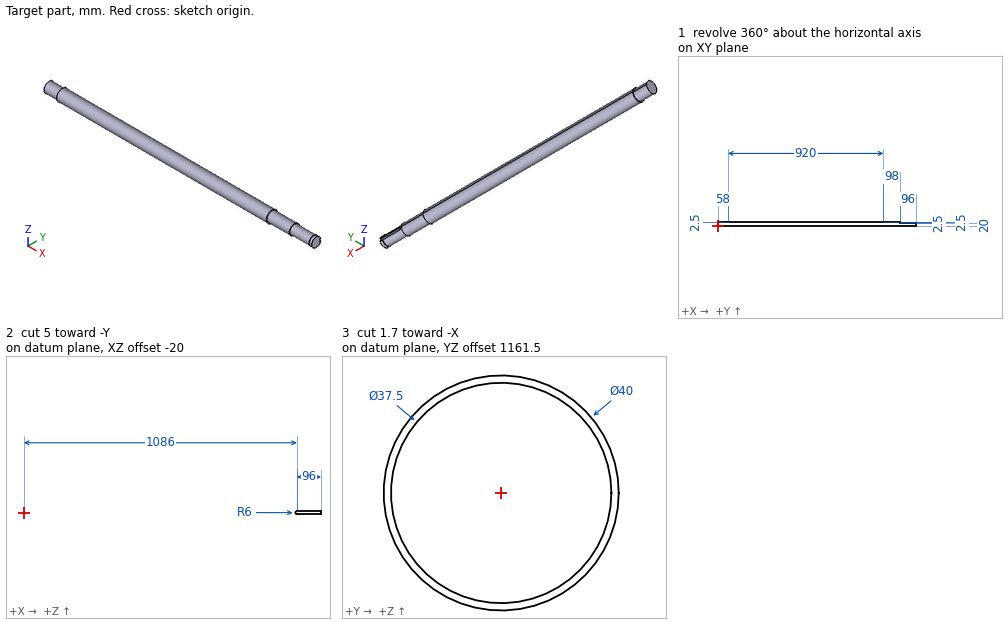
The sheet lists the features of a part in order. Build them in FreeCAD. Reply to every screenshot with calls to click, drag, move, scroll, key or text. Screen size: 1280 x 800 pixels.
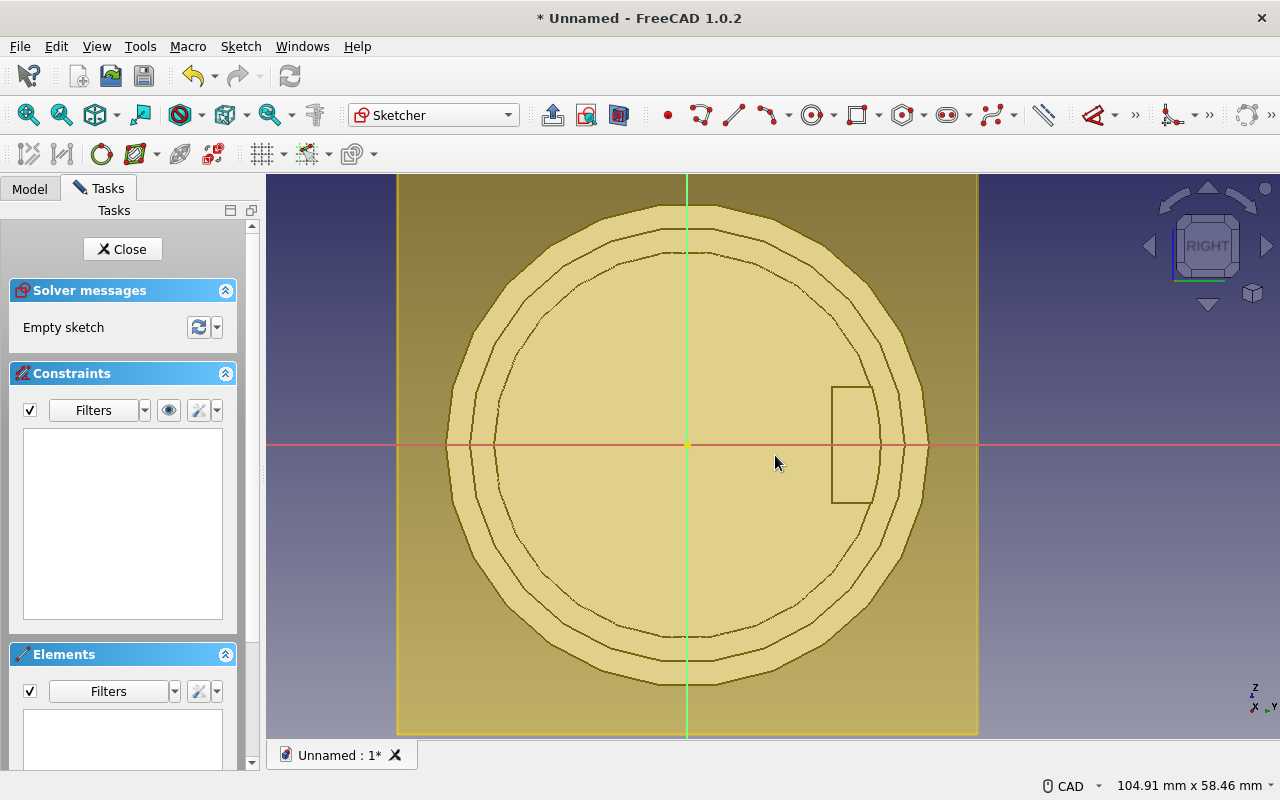
click(812, 116)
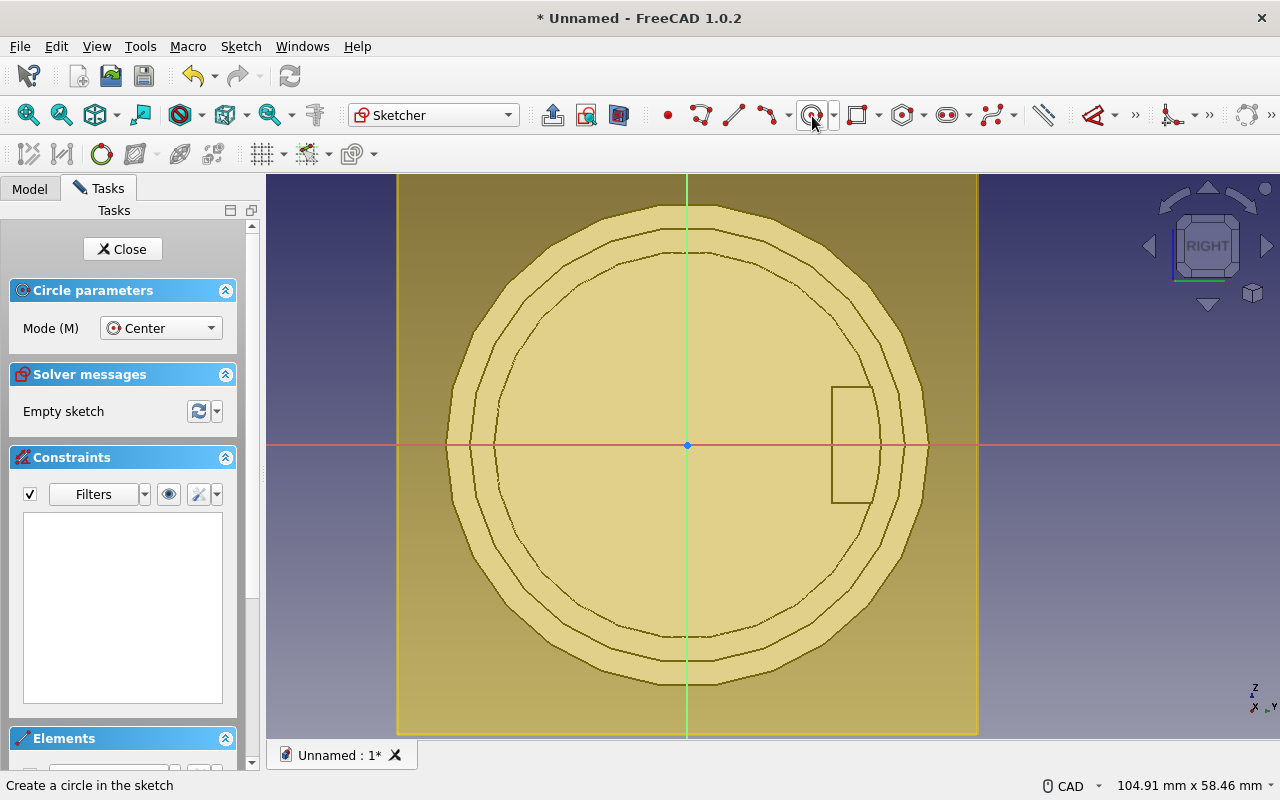
click(687, 445)
click(824, 308)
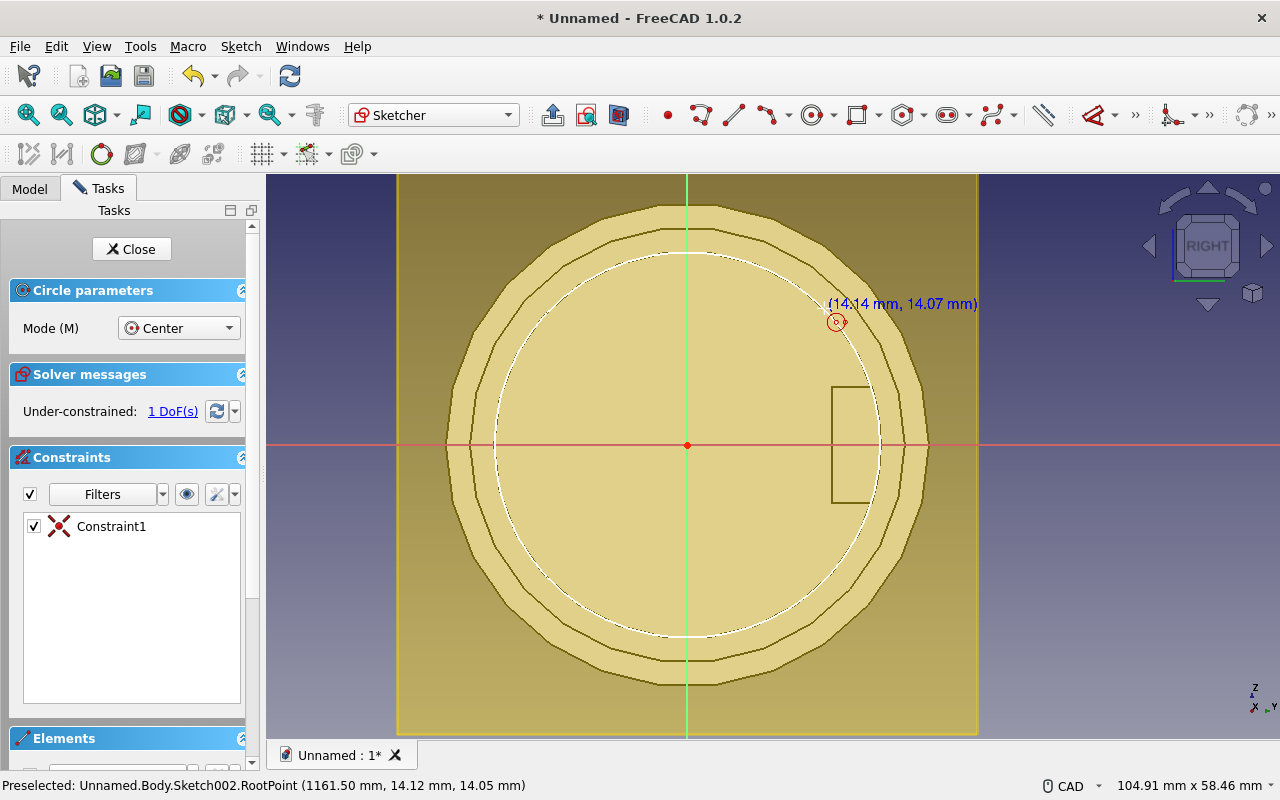
click(687, 445)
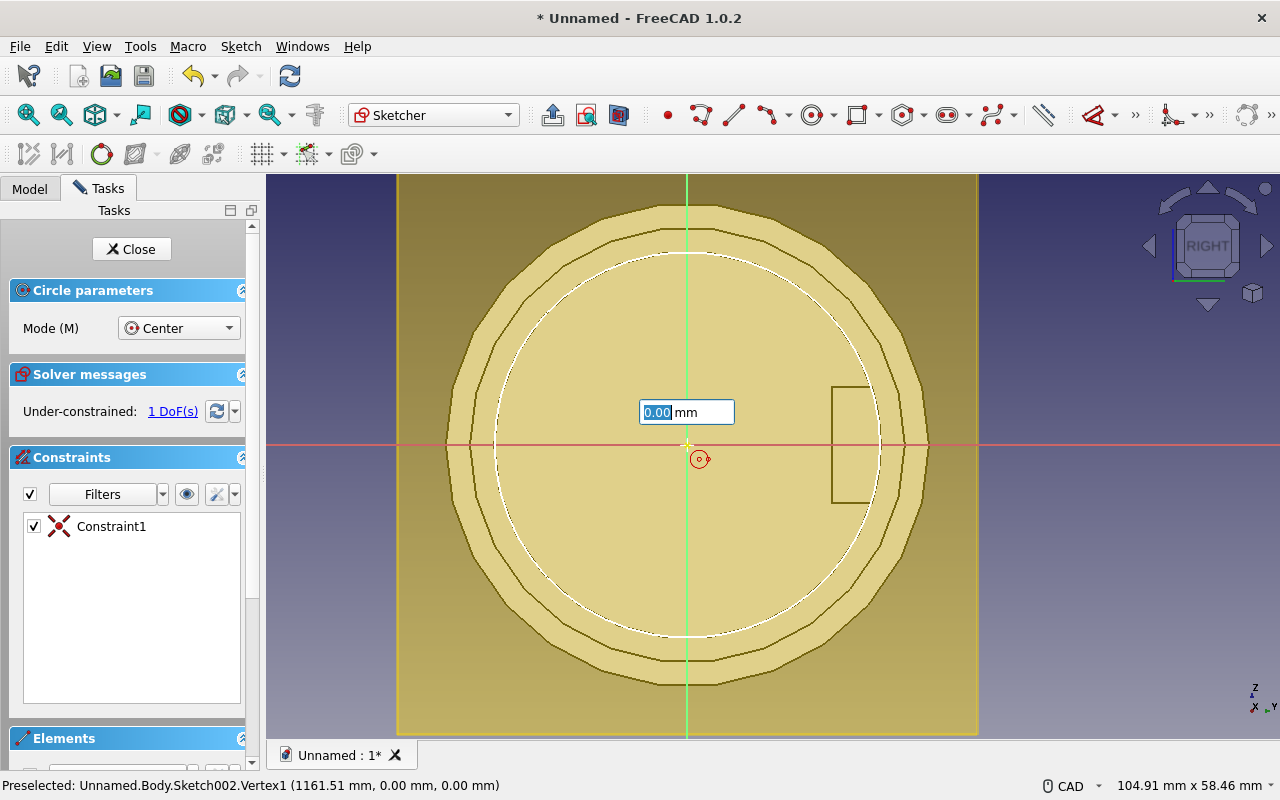
scroll(816, 317, up, 2)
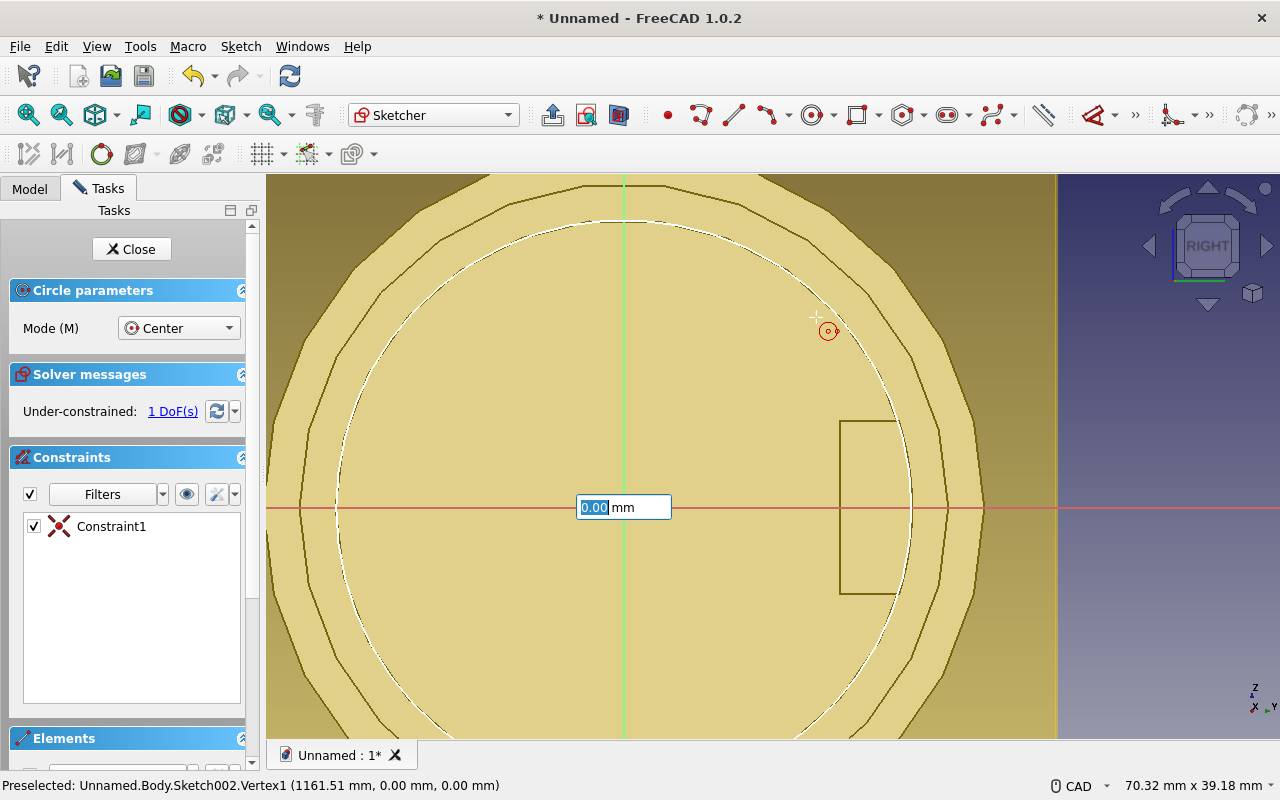
click(815, 317)
key(Escape)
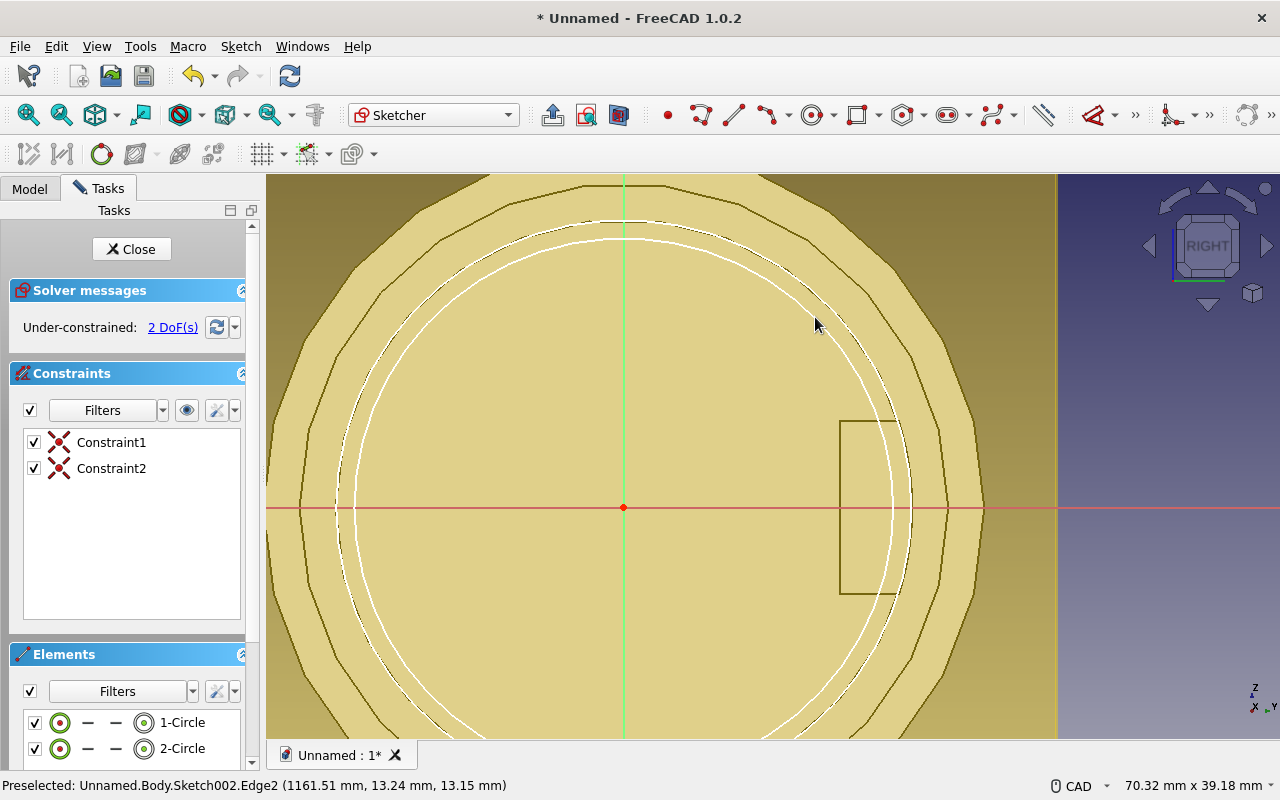
click(1092, 116)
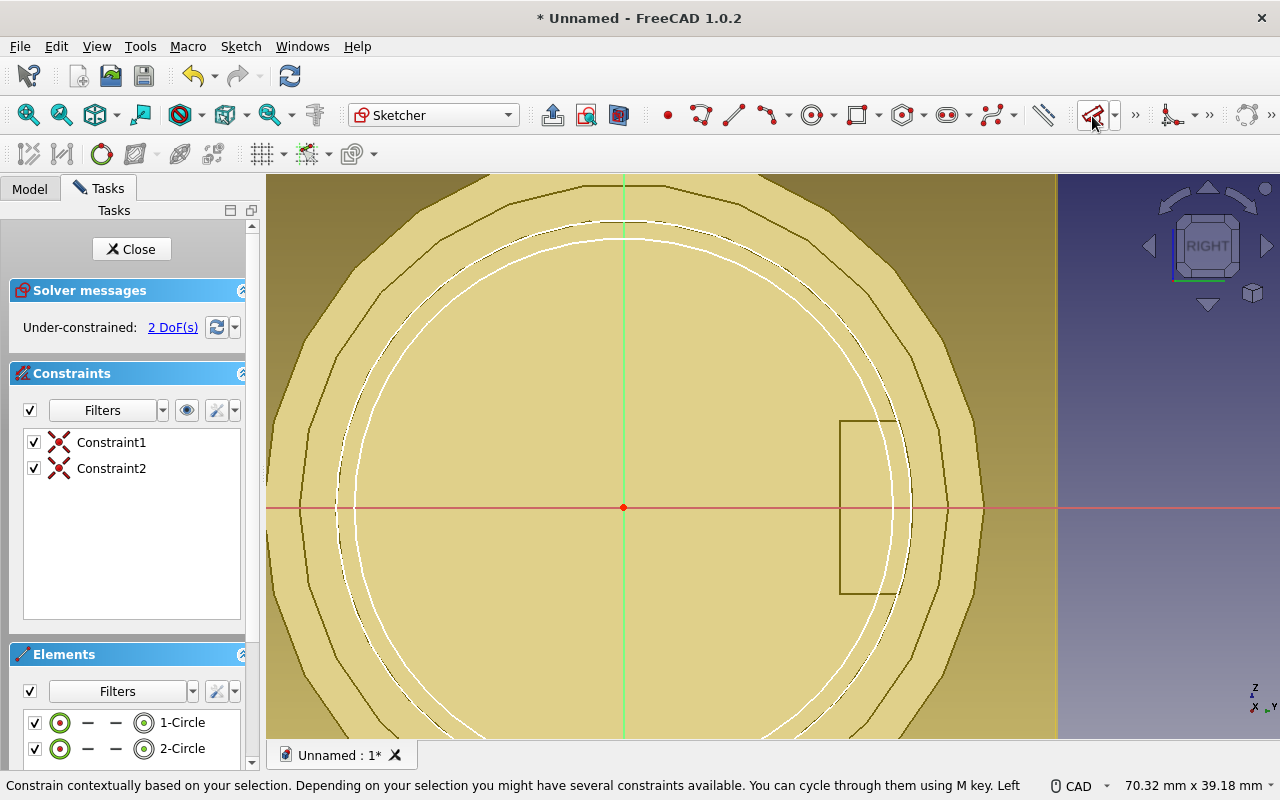
click(827, 304)
click(850, 281)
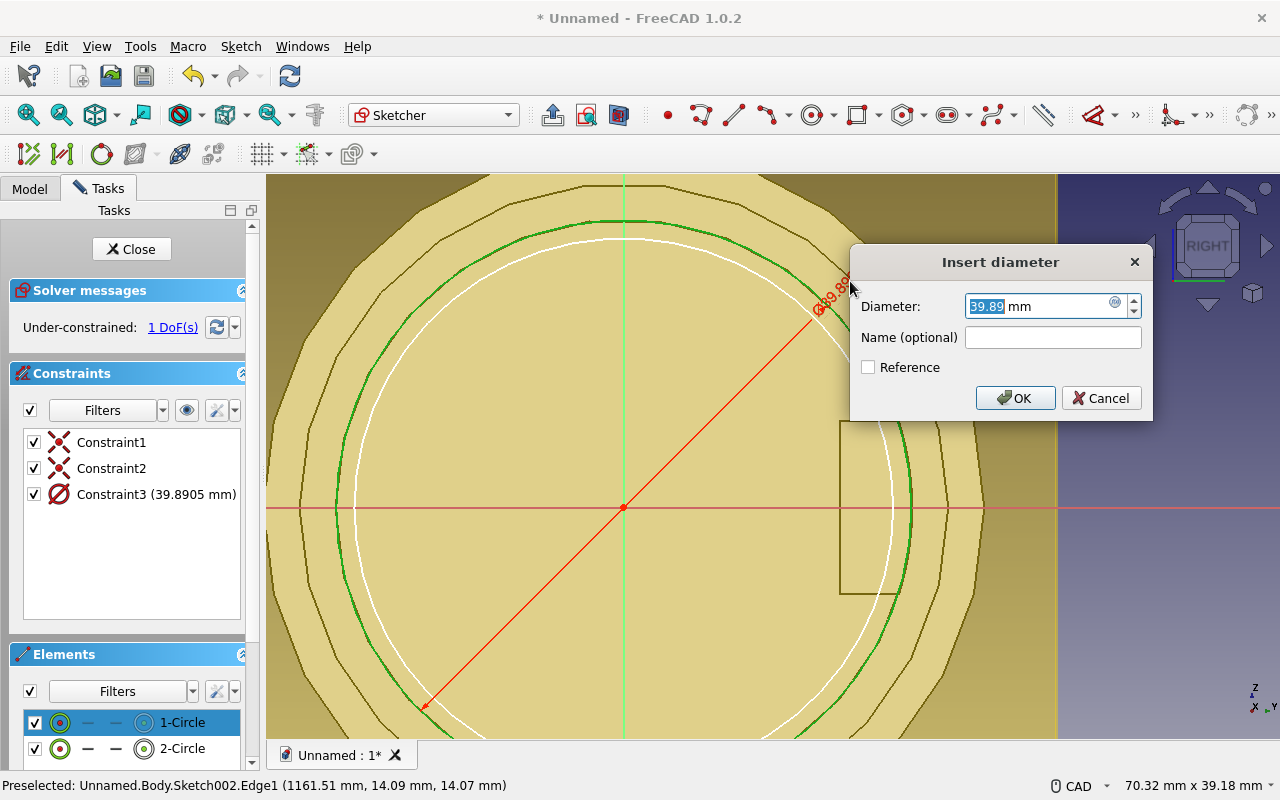
text(40)
key(Return)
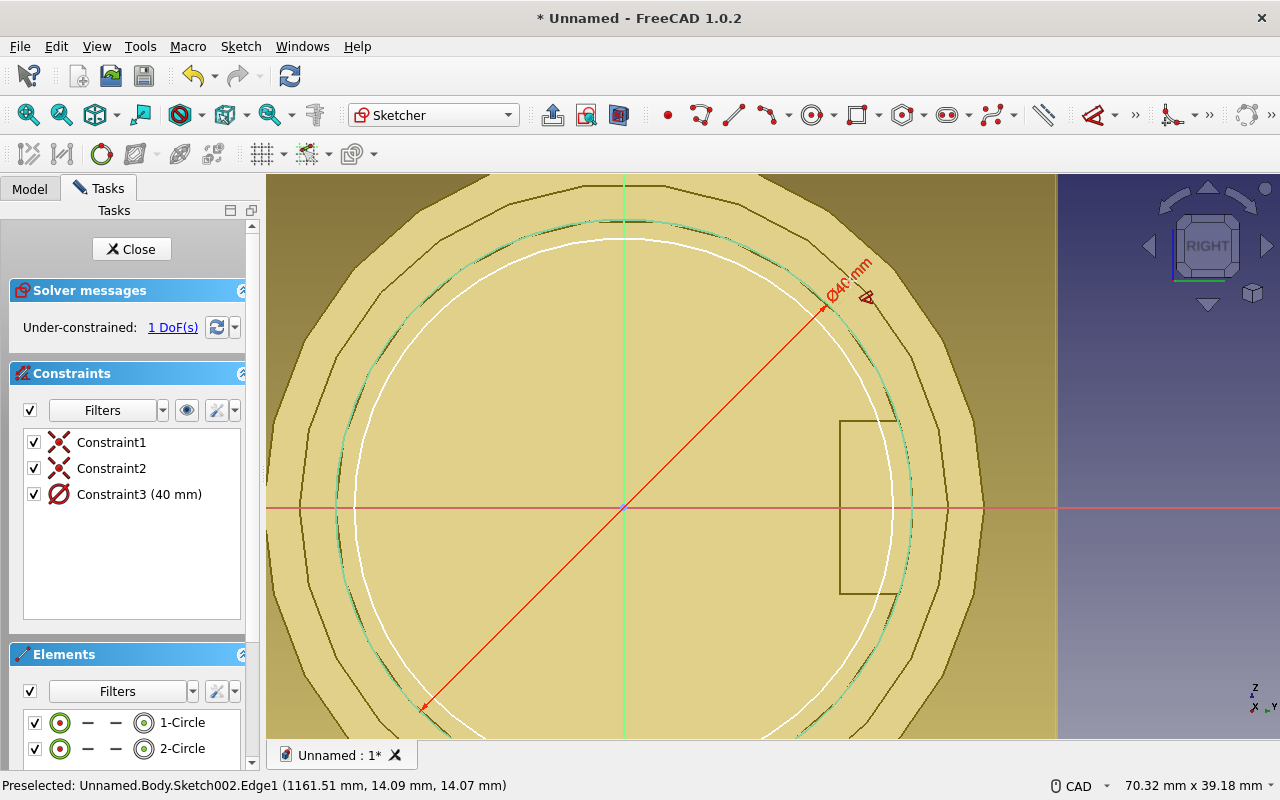
click(814, 317)
click(913, 422)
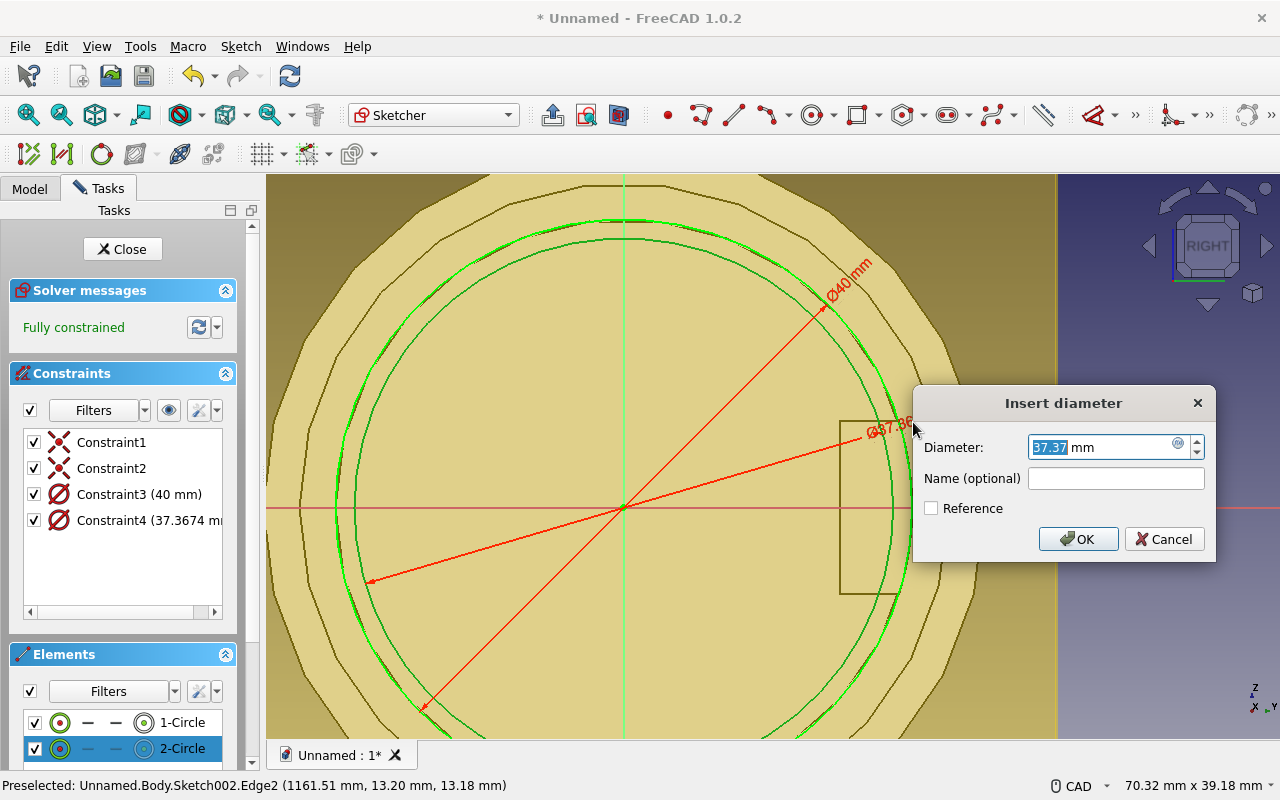
text(37.5)
key(Return)
key(Escape)